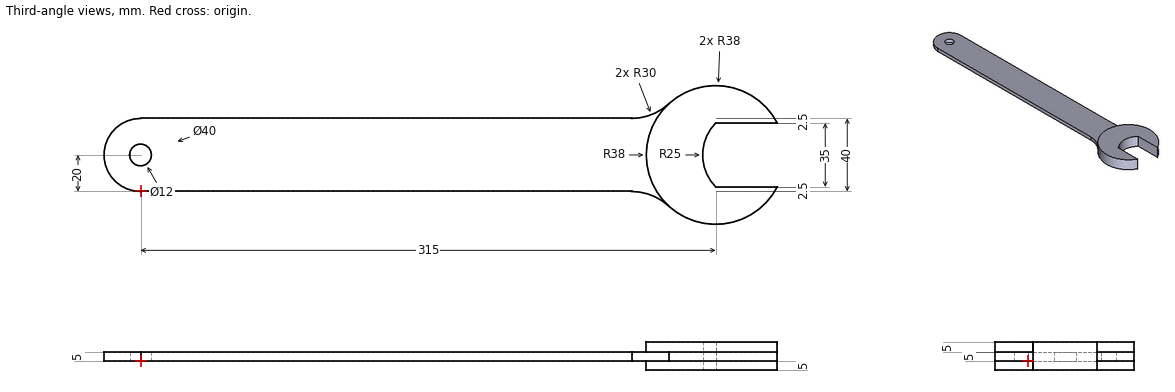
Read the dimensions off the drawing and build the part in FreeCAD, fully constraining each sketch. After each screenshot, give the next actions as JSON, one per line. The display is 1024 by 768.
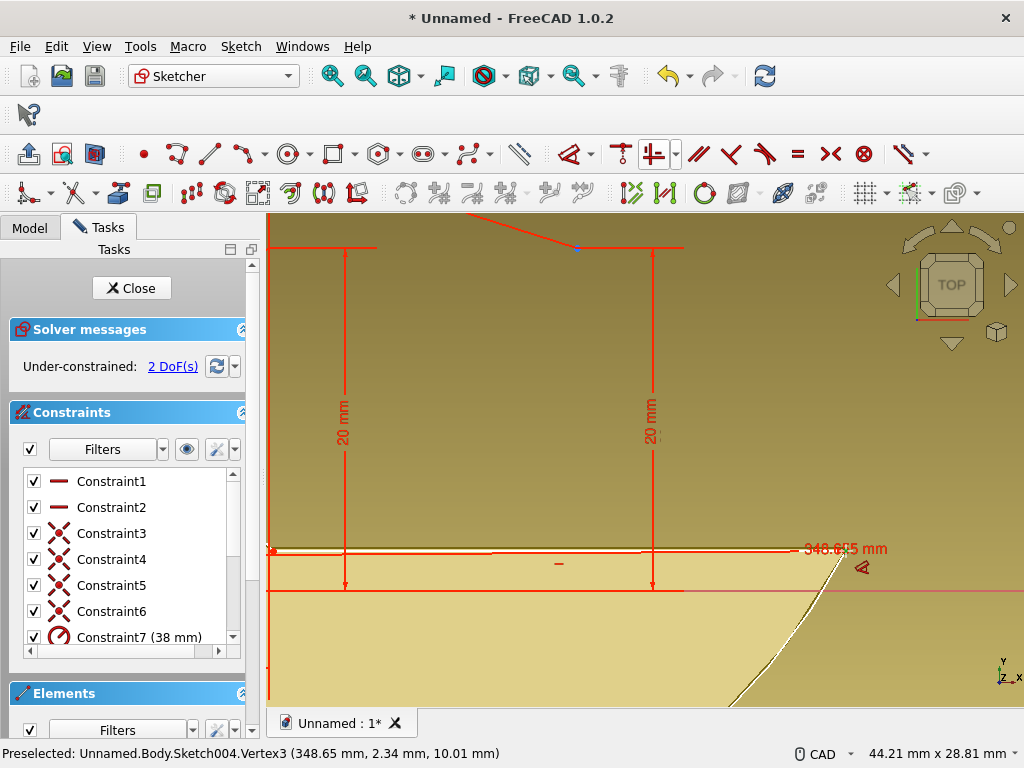
{"action": "key", "text": "Escape"}
{"action": "key", "text": "Escape"}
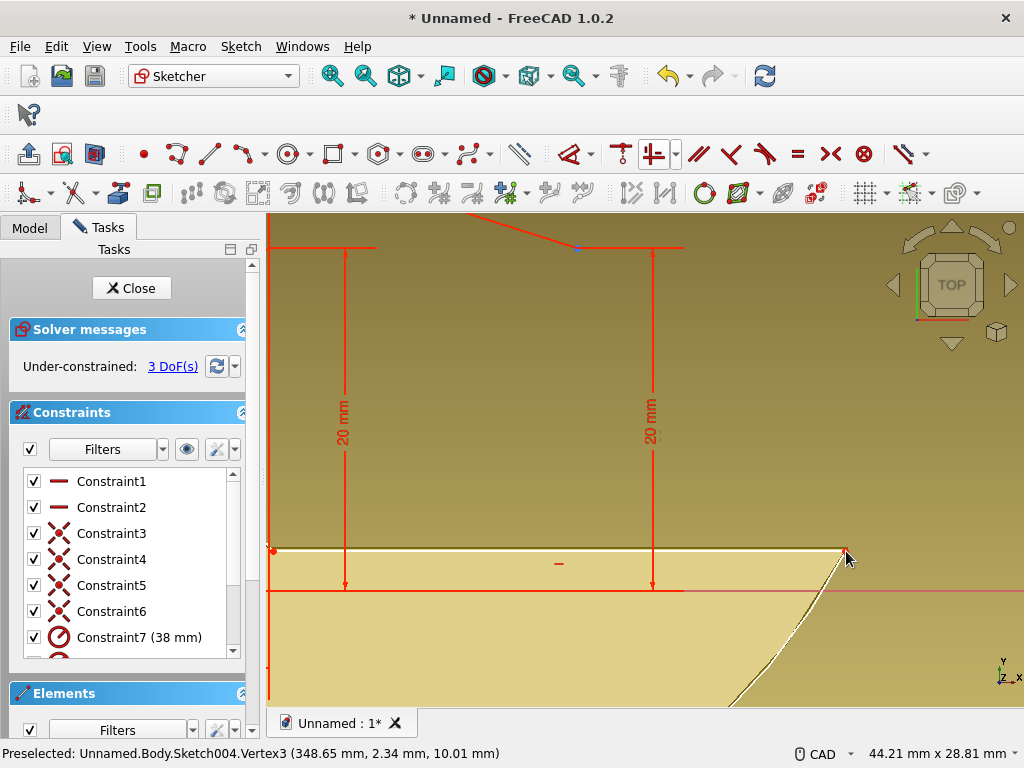
{"action": "left_click", "coordinate": [846, 551]}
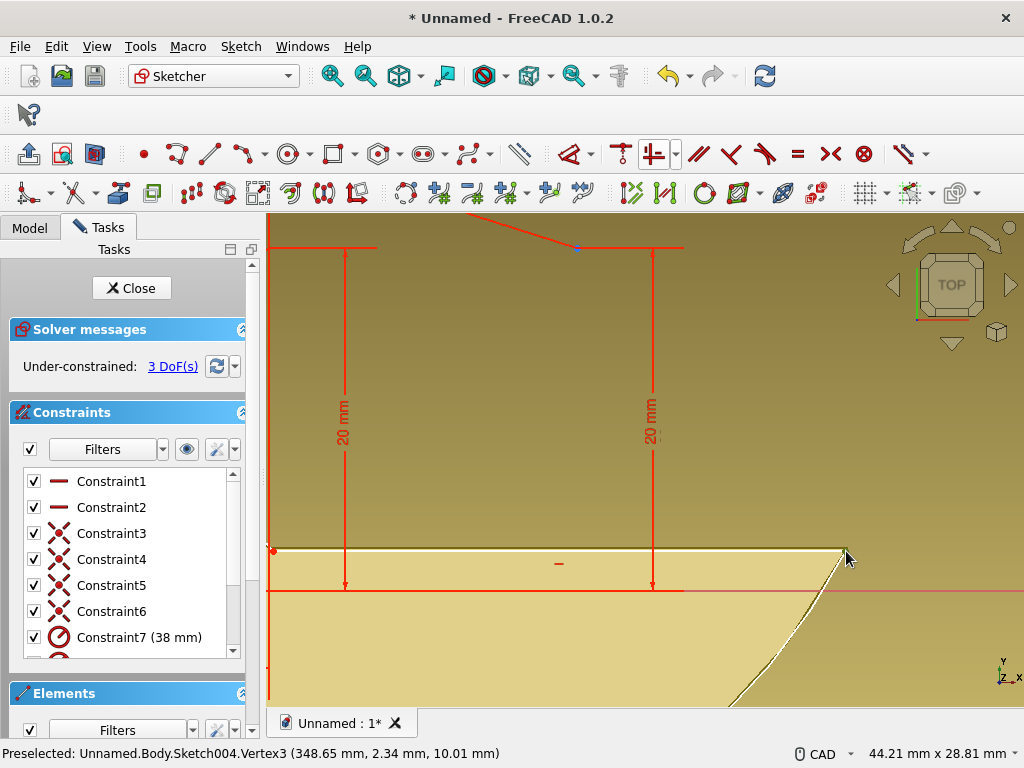
{"action": "left_click", "coordinate": [590, 154]}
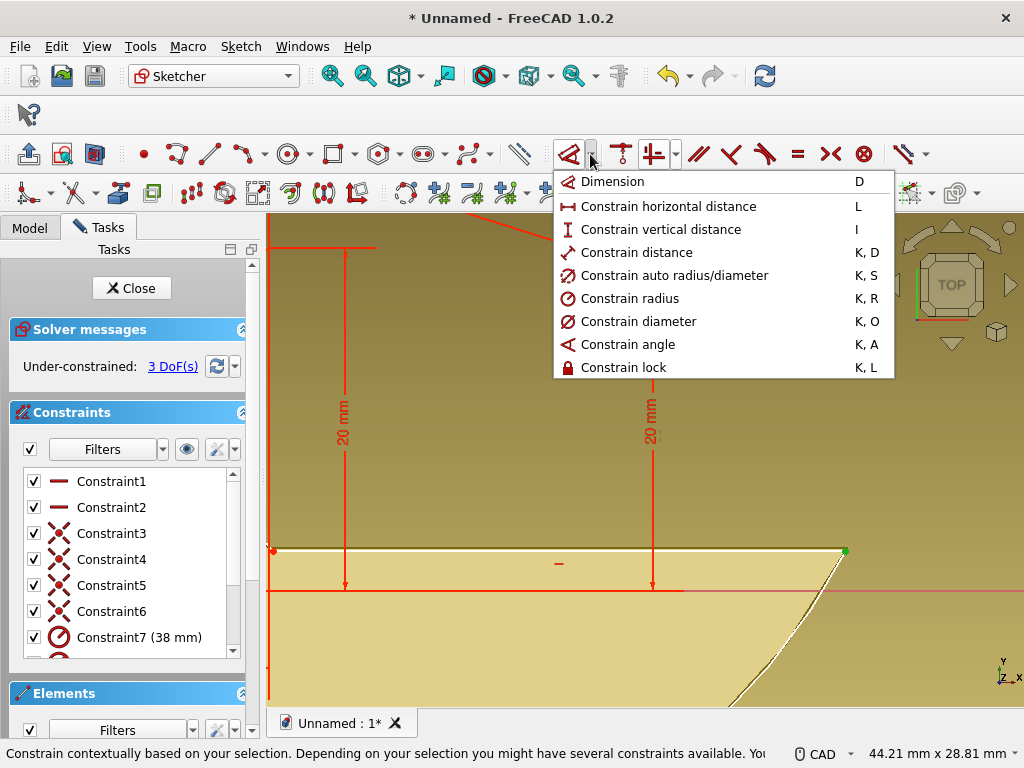
{"action": "left_click", "coordinate": [724, 230]}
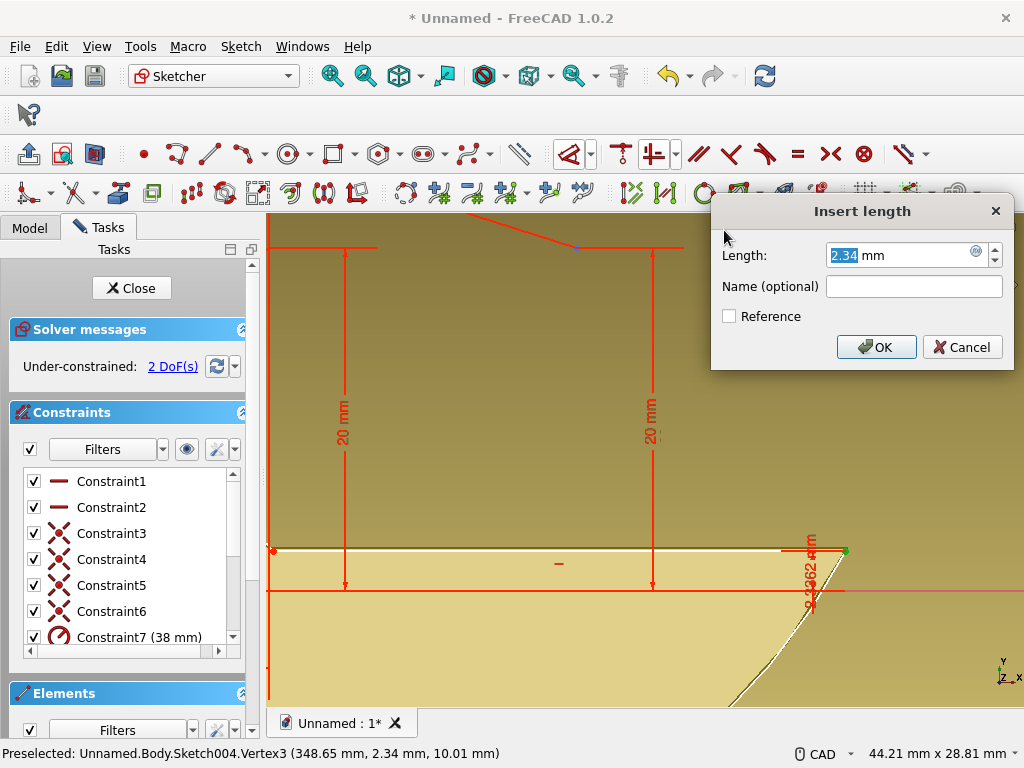
{"action": "type", "text": "2.5"}
{"action": "key", "text": "Return"}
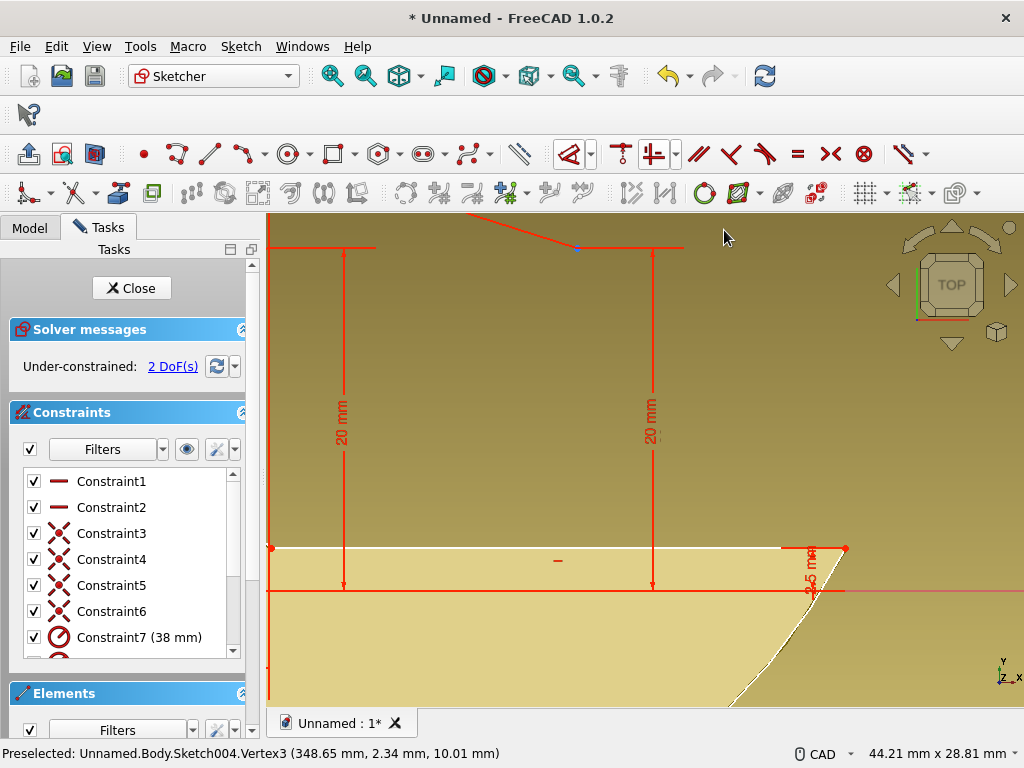
{"action": "scroll", "coordinate": [725, 551], "scroll_direction": "down", "scroll_amount": 6}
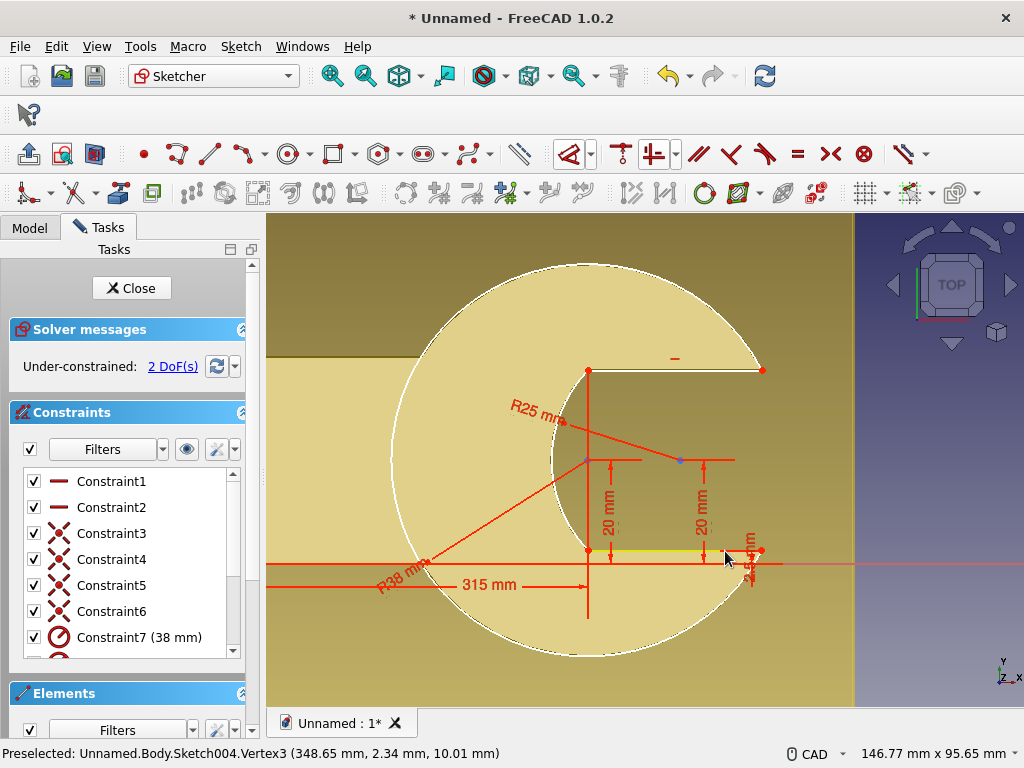
{"action": "left_click", "coordinate": [589, 551]}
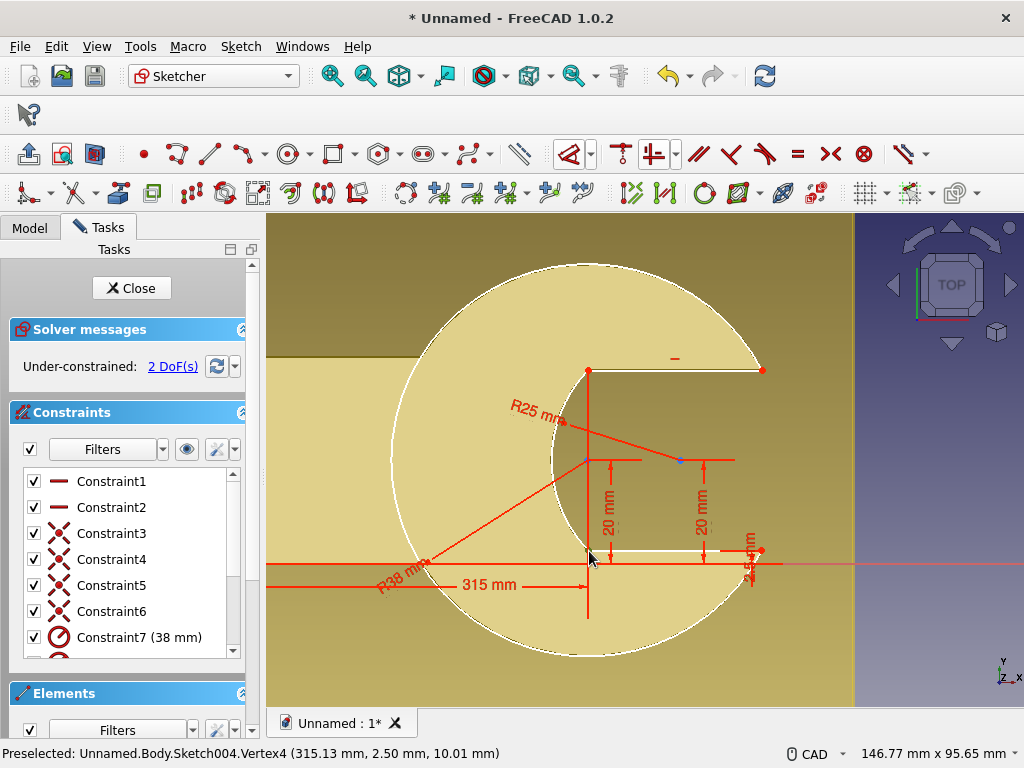
{"action": "left_click", "coordinate": [590, 154]}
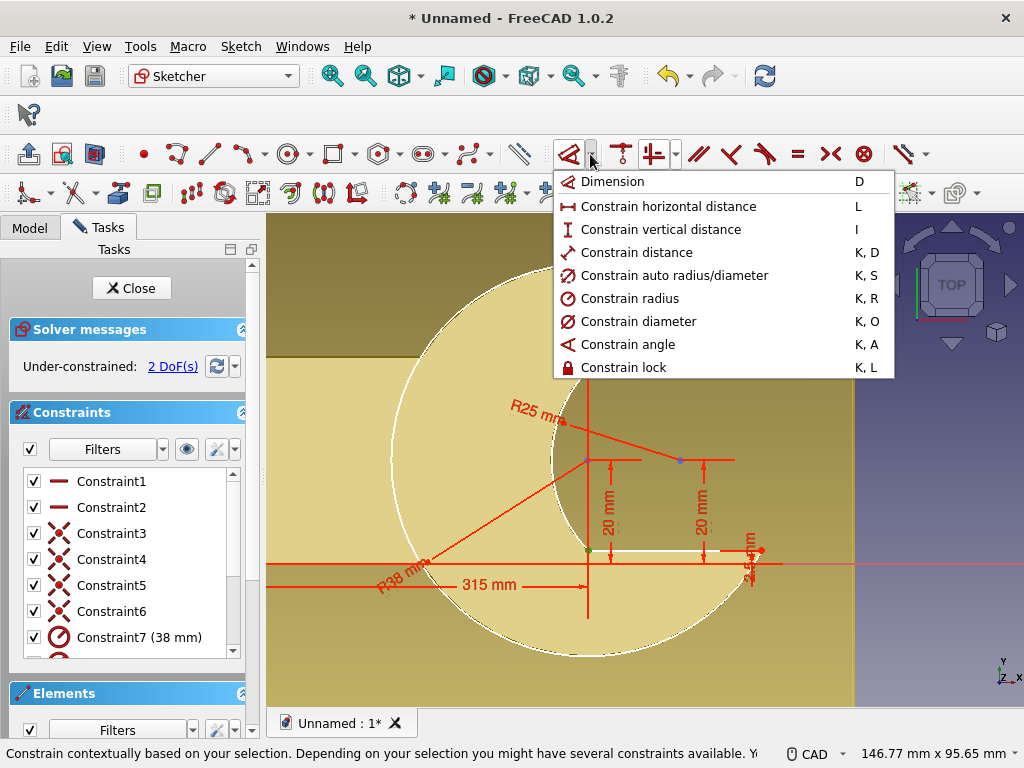
{"action": "left_click", "coordinate": [724, 206]}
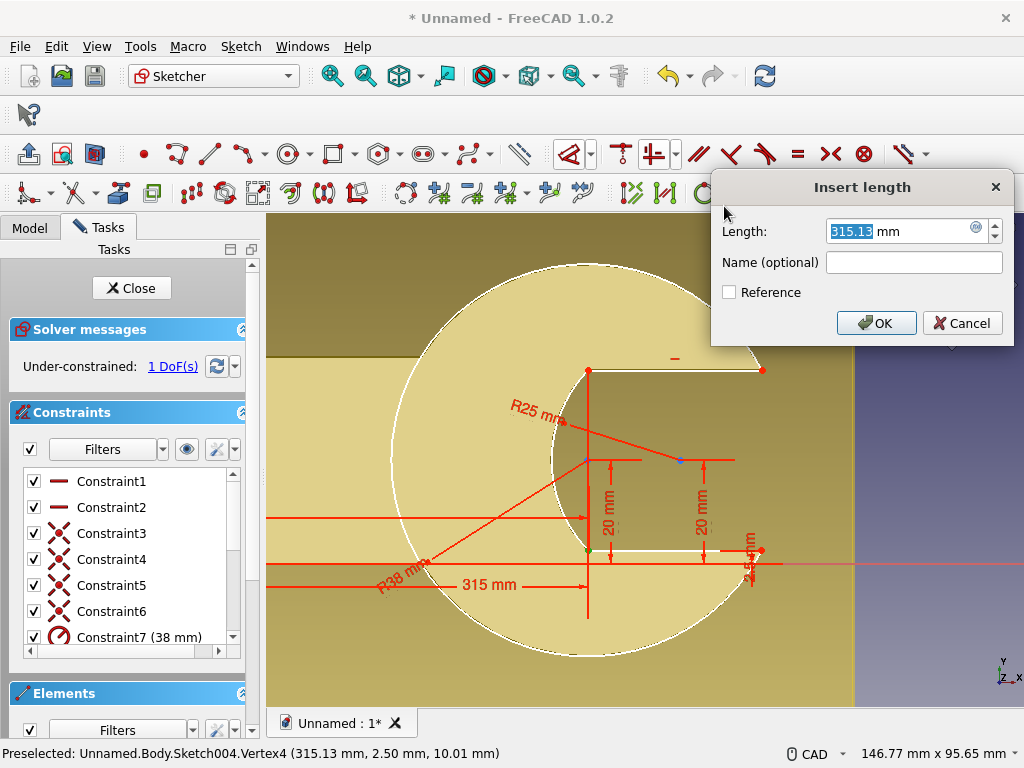
{"action": "type", "text": "315"}
{"action": "key", "text": "Return"}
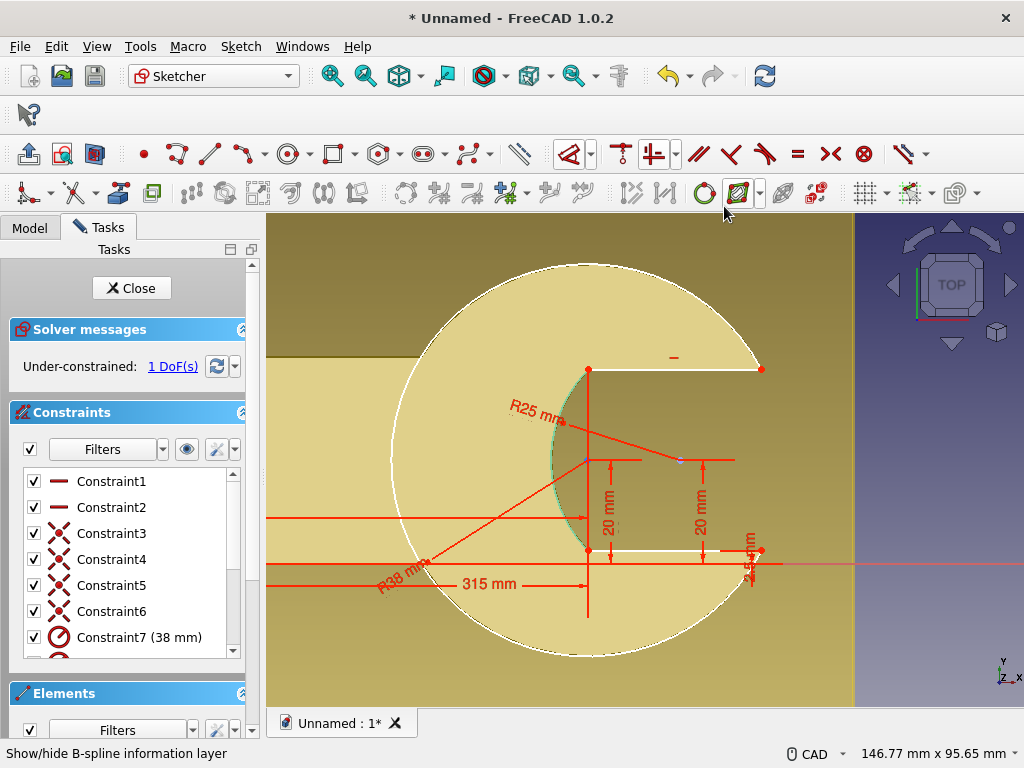
{"action": "left_click", "coordinate": [588, 460]}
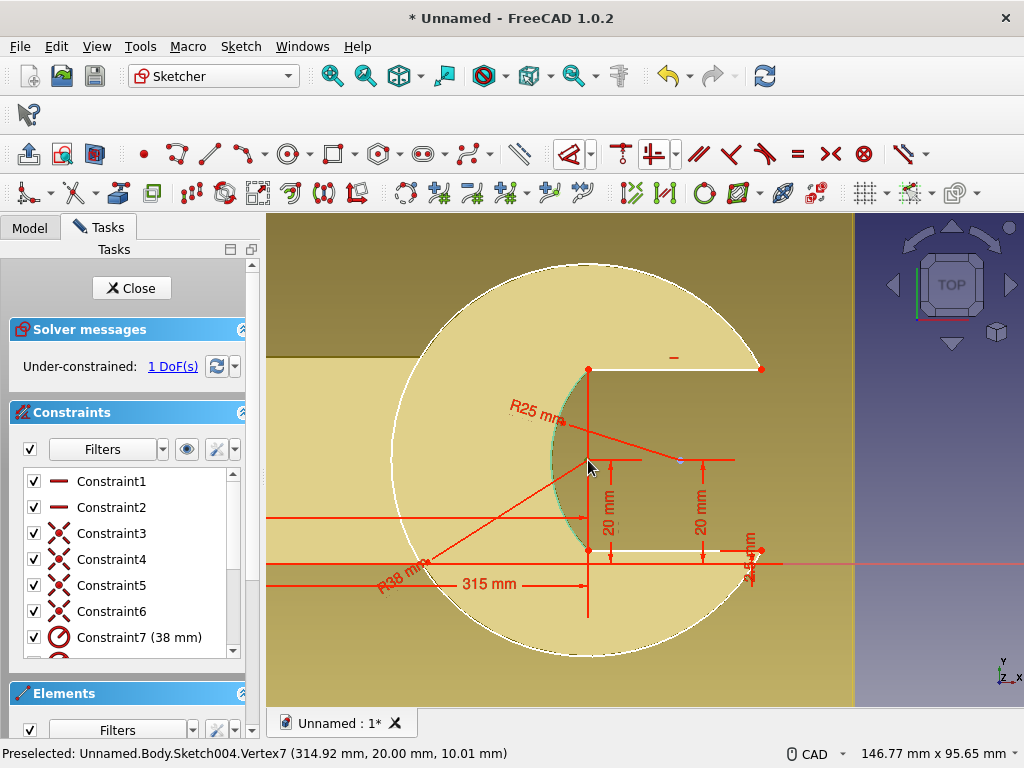
{"action": "key", "text": "l"}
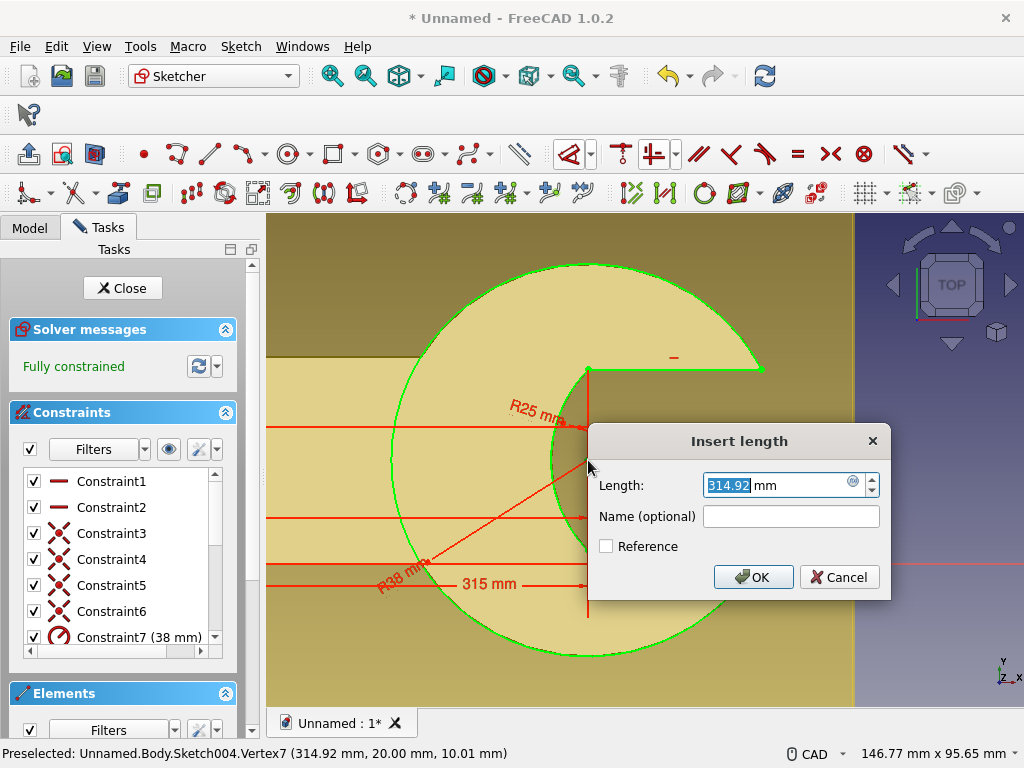
{"action": "type", "text": "315"}
{"action": "key", "text": "Return"}